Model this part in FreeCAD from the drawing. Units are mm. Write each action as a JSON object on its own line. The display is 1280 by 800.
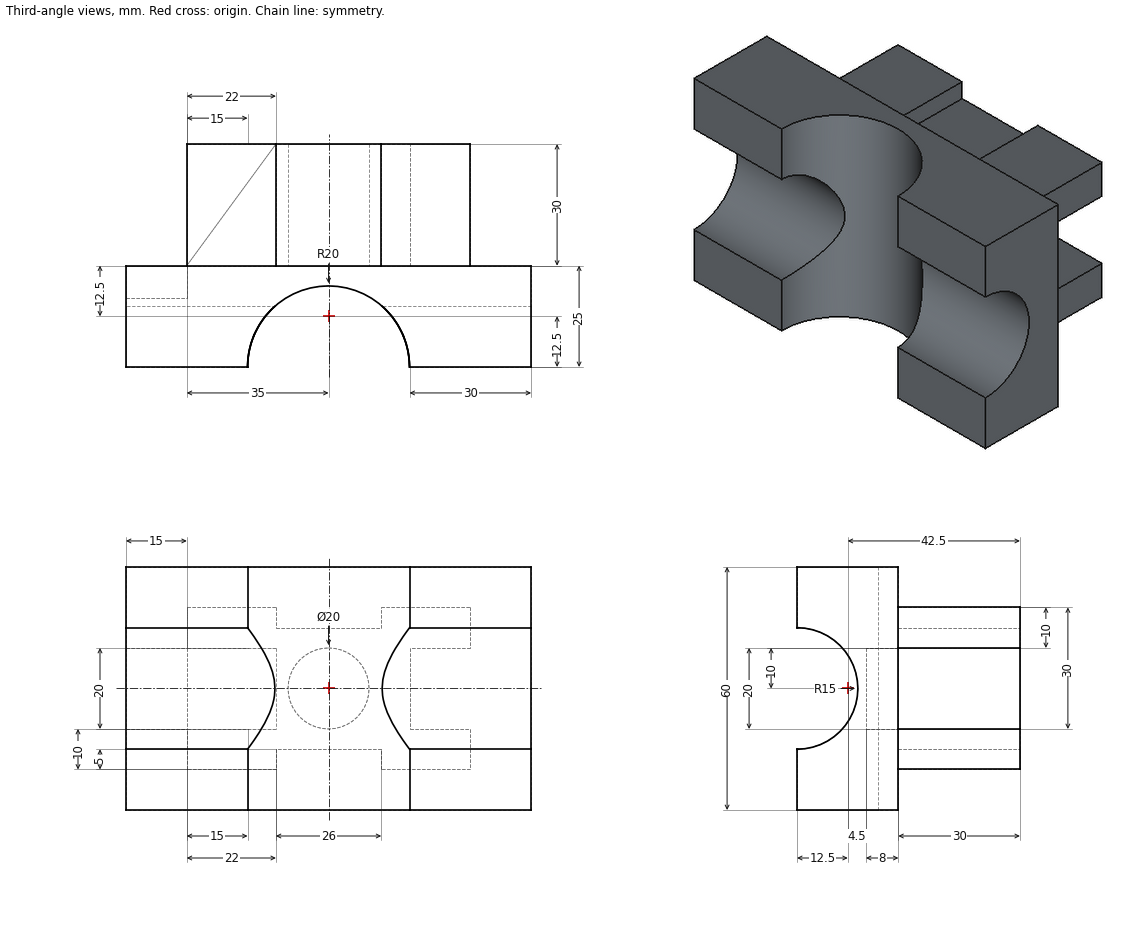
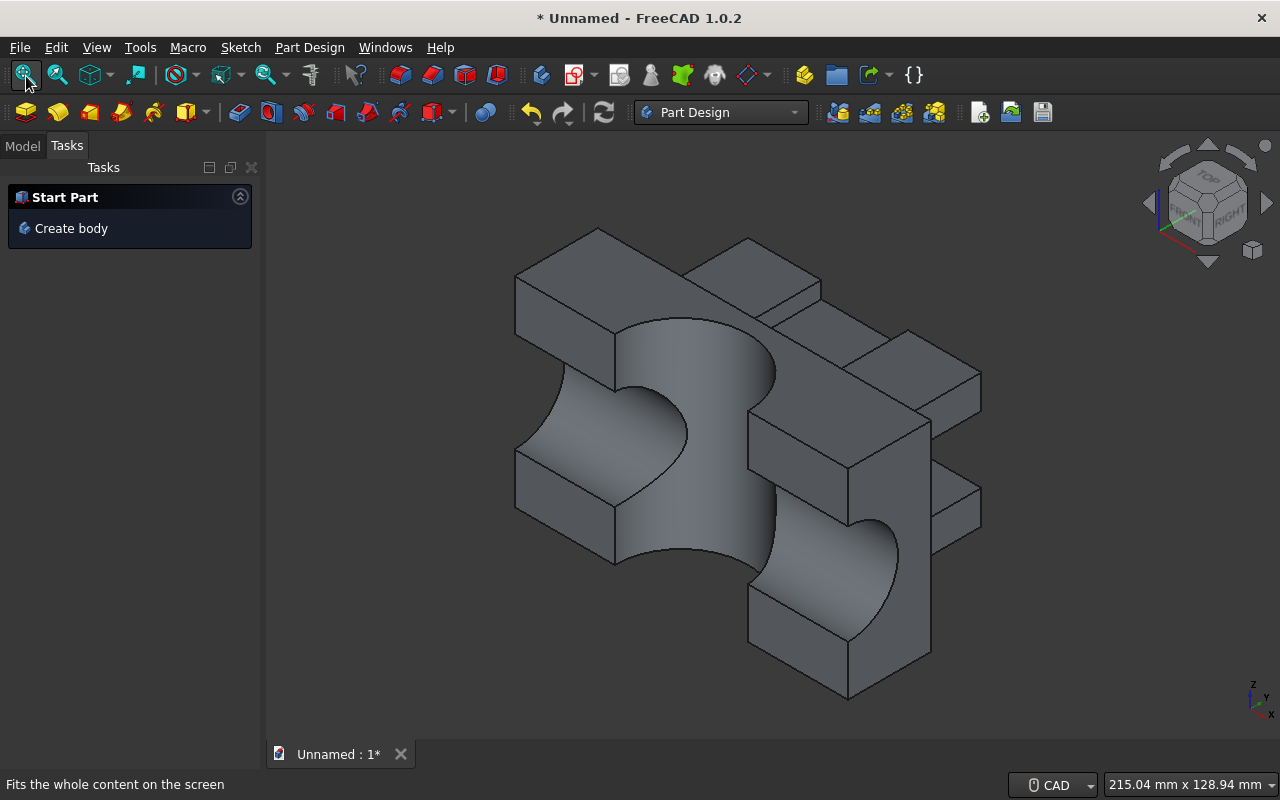
{"action": "left_click", "coordinate": [735, 287]}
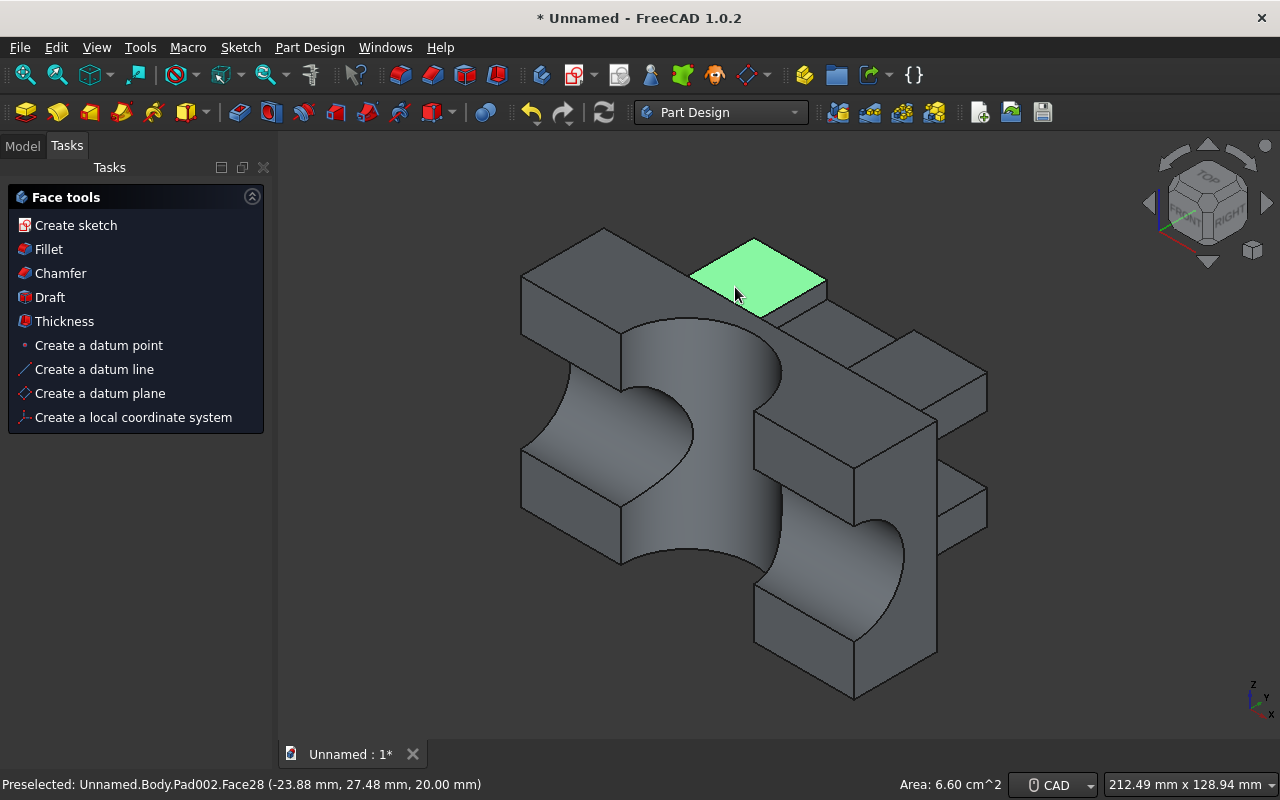
{"action": "left_click", "coordinate": [574, 76]}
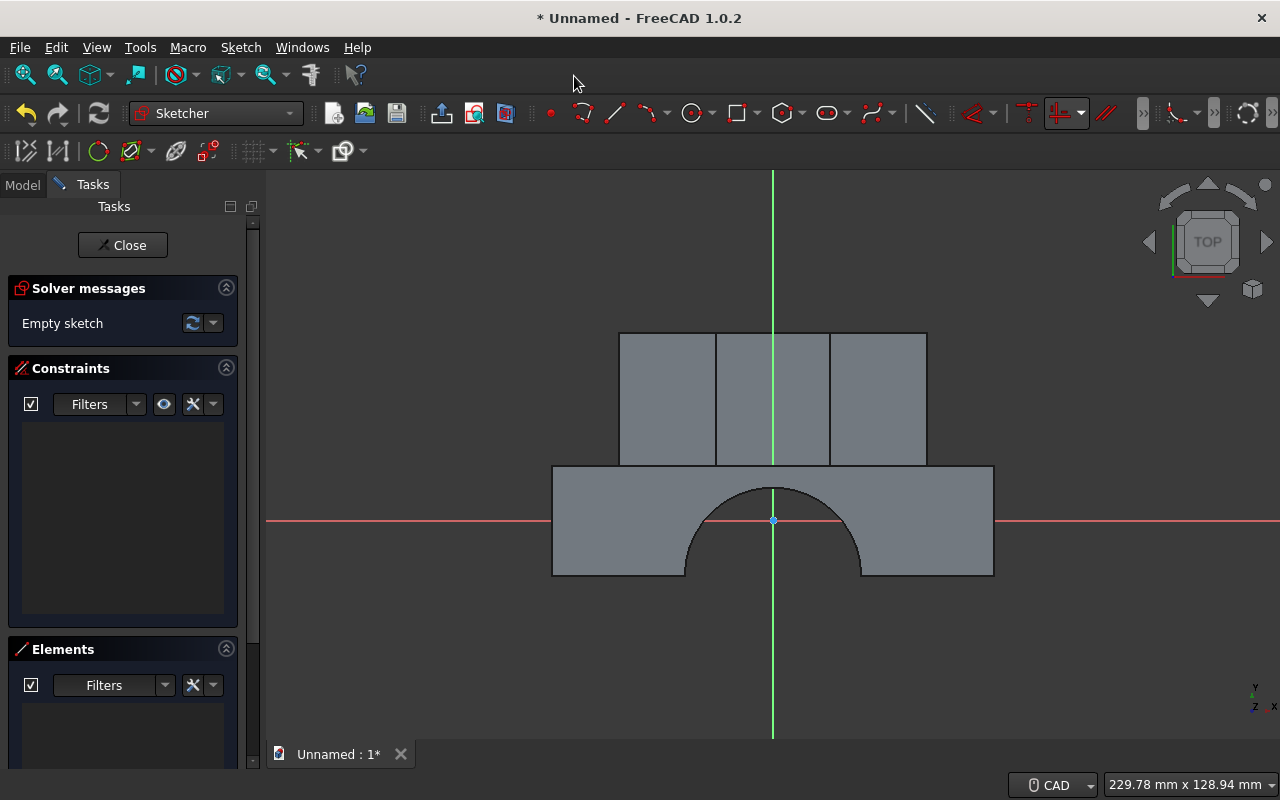
{"action": "key", "text": "q s"}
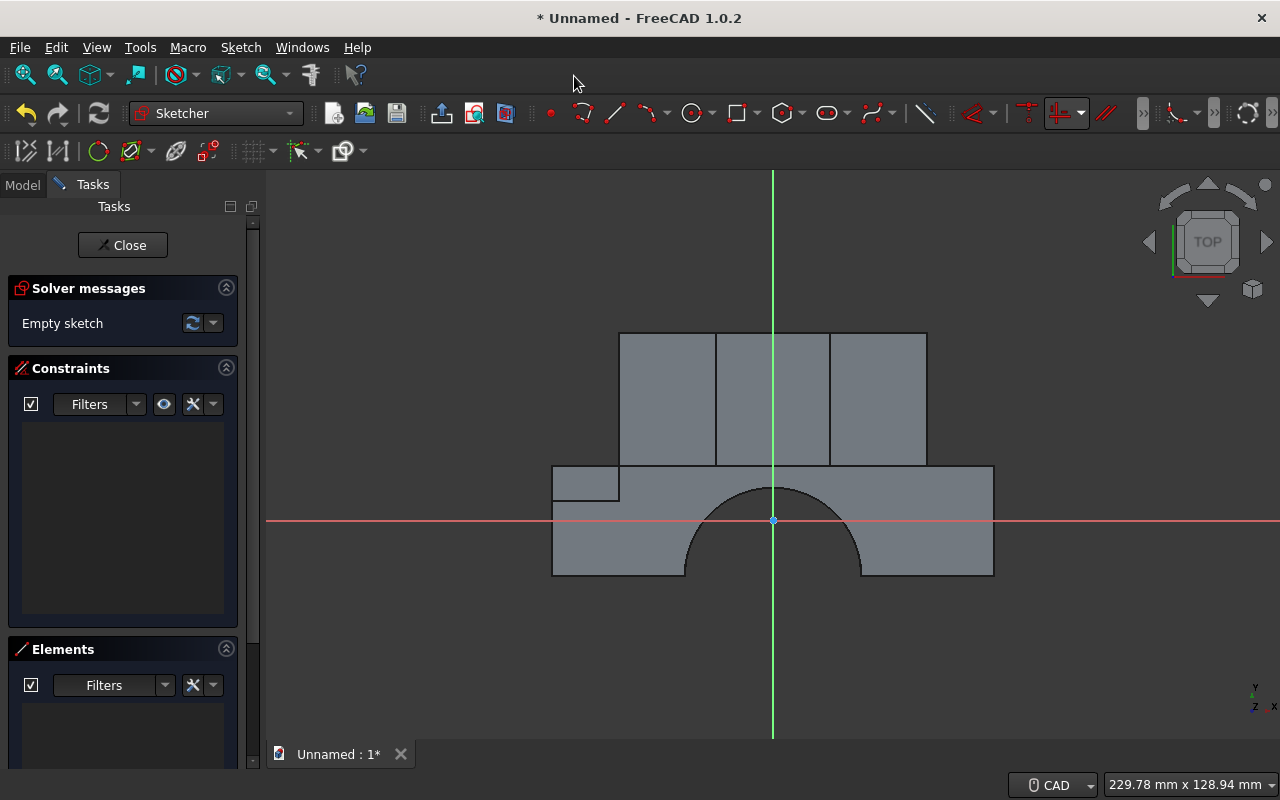
{"action": "scroll", "coordinate": [685, 393], "scroll_direction": "up", "scroll_amount": 3}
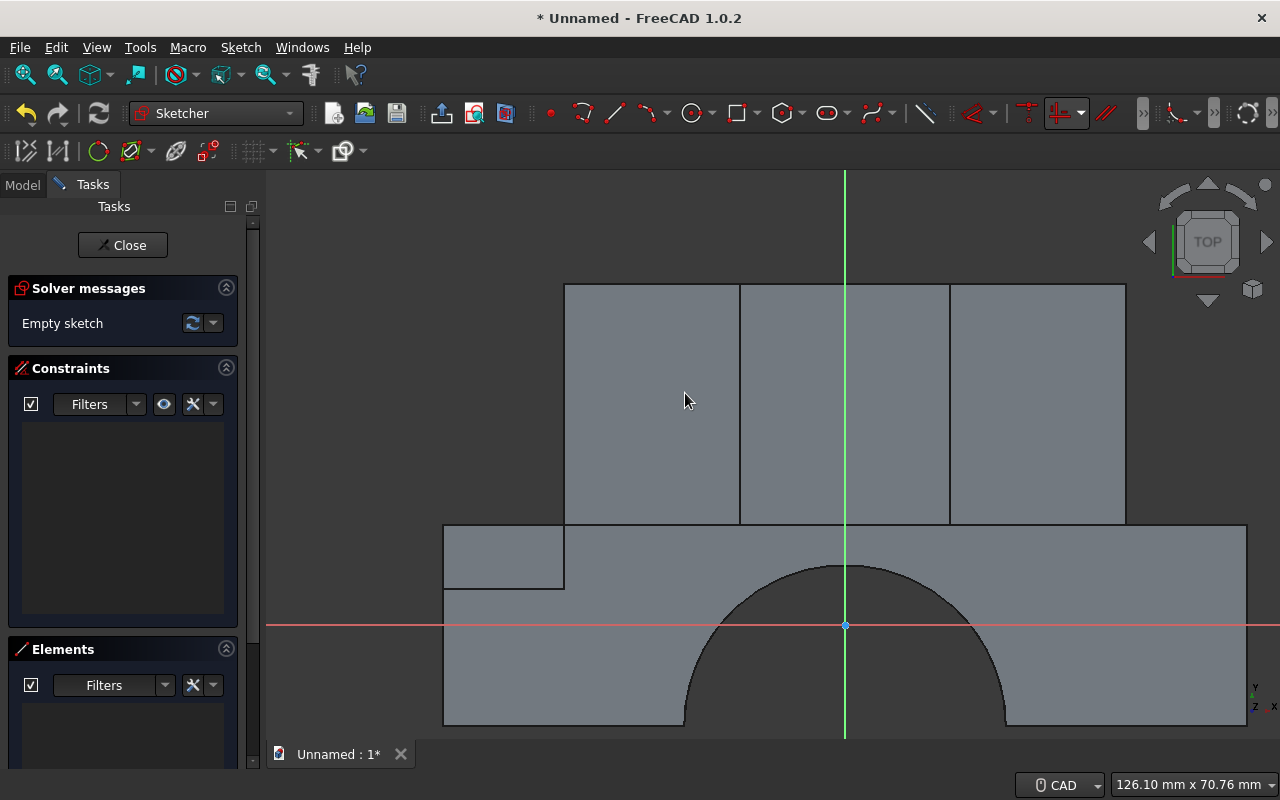
{"action": "left_click", "coordinate": [584, 114]}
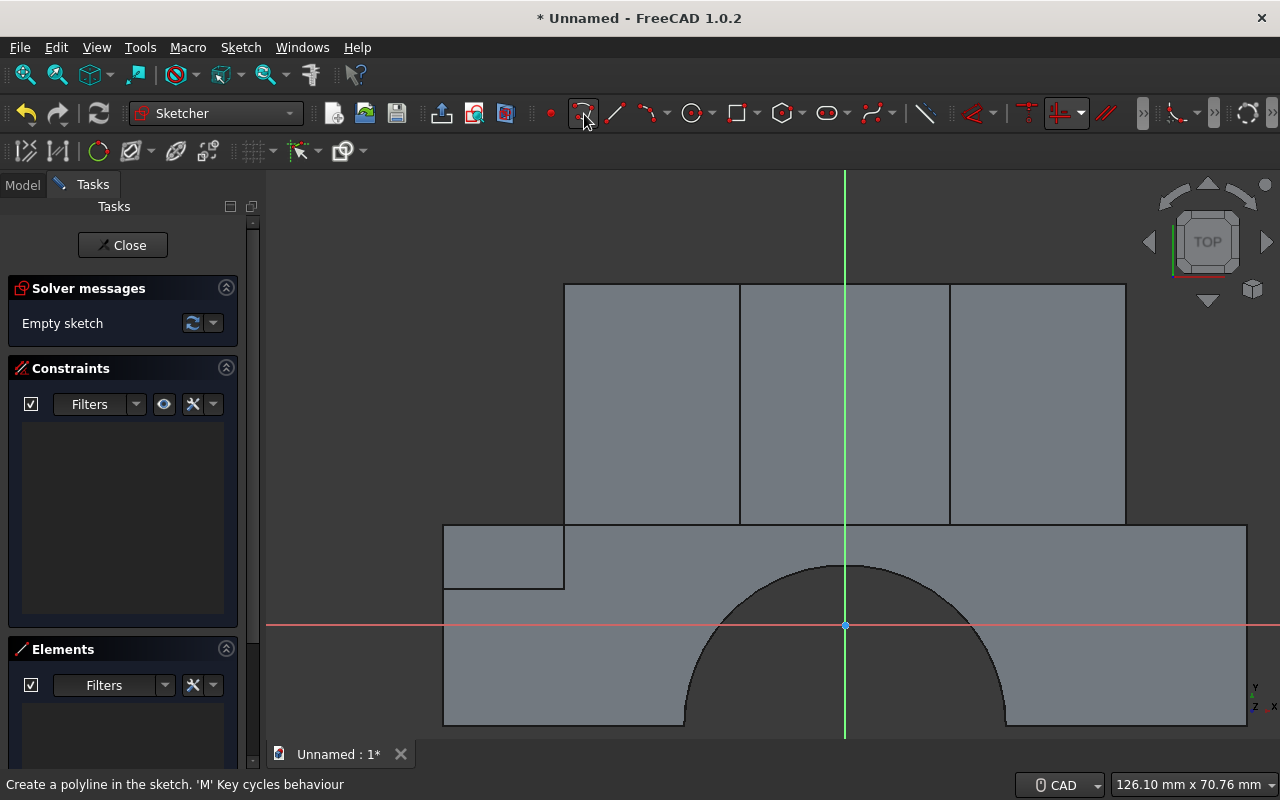
{"action": "left_click", "coordinate": [564, 525]}
{"action": "left_click", "coordinate": [740, 284]}
{"action": "left_click", "coordinate": [564, 284]}
{"action": "left_click", "coordinate": [564, 526]}
{"action": "key", "text": "Escape"}
{"action": "key", "text": "Escape"}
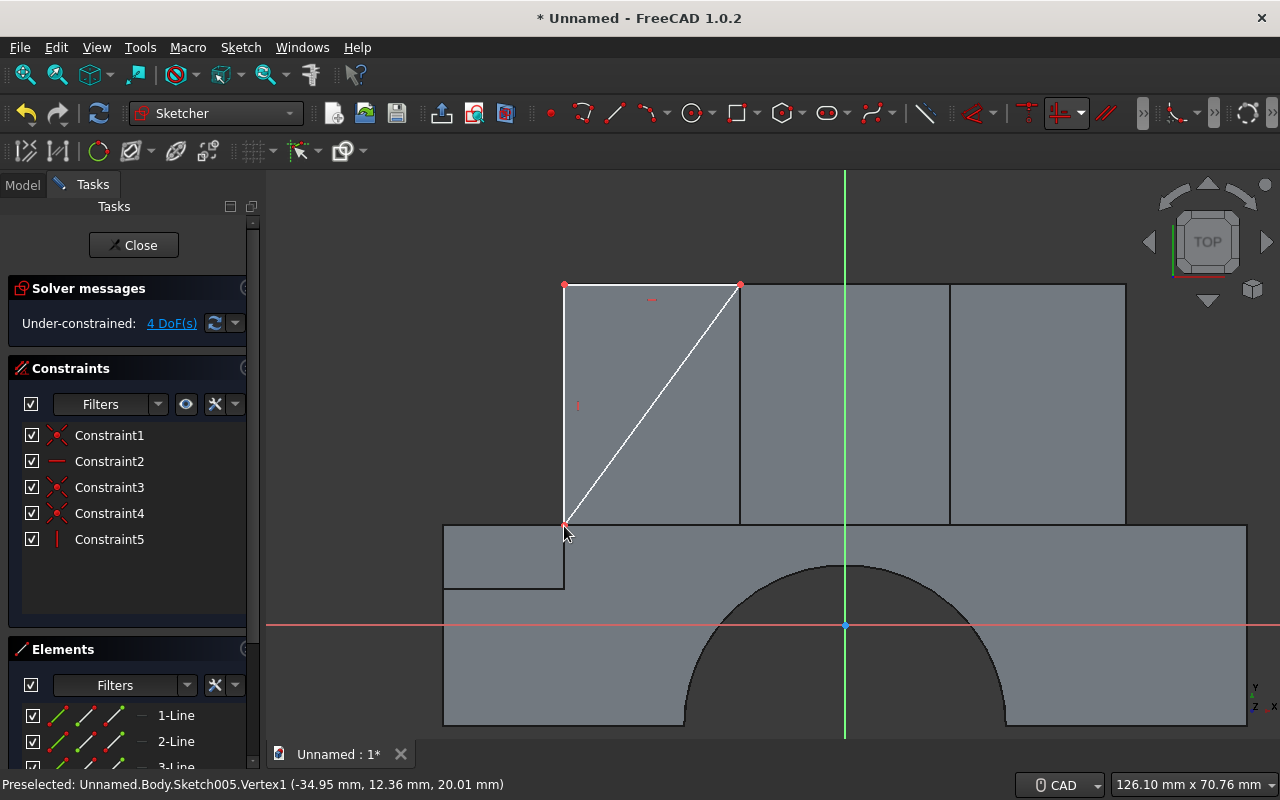
{"action": "left_click", "coordinate": [972, 114]}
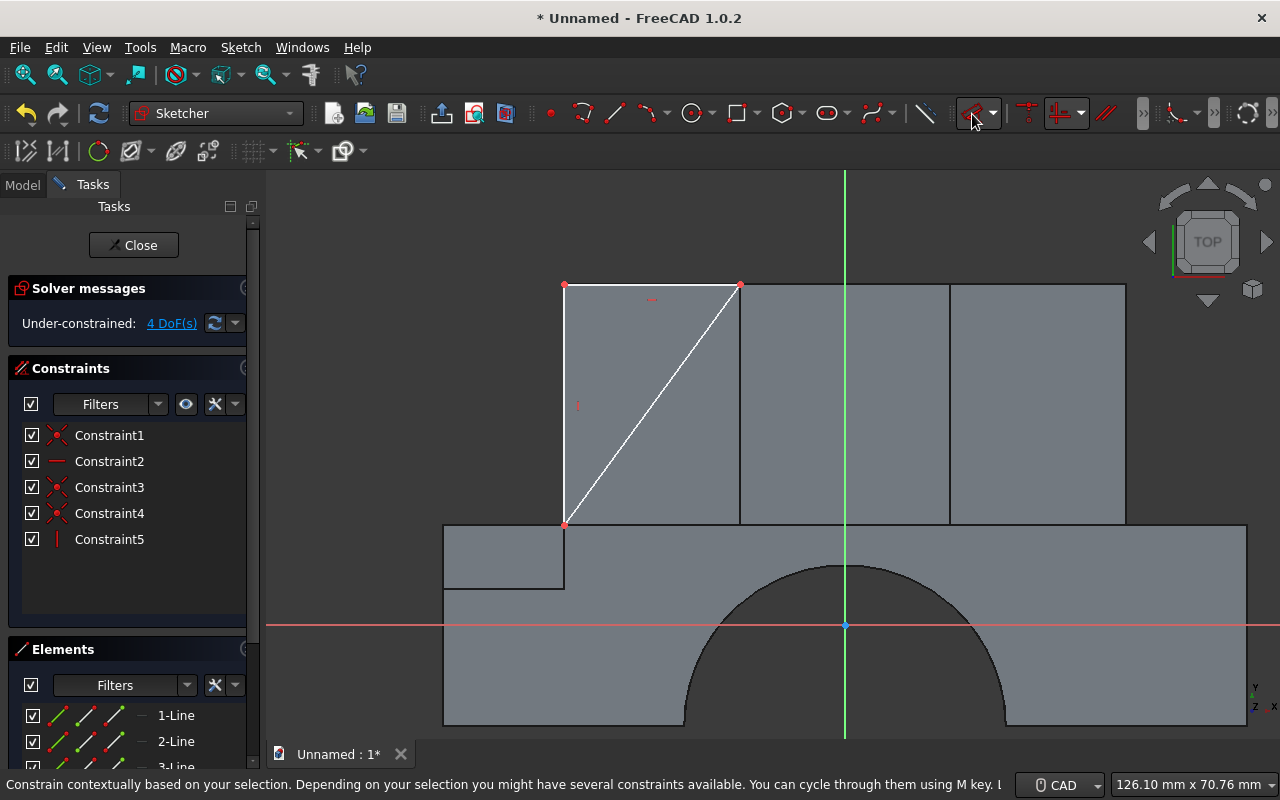
{"action": "left_click", "coordinate": [687, 285]}
{"action": "left_click", "coordinate": [652, 251]}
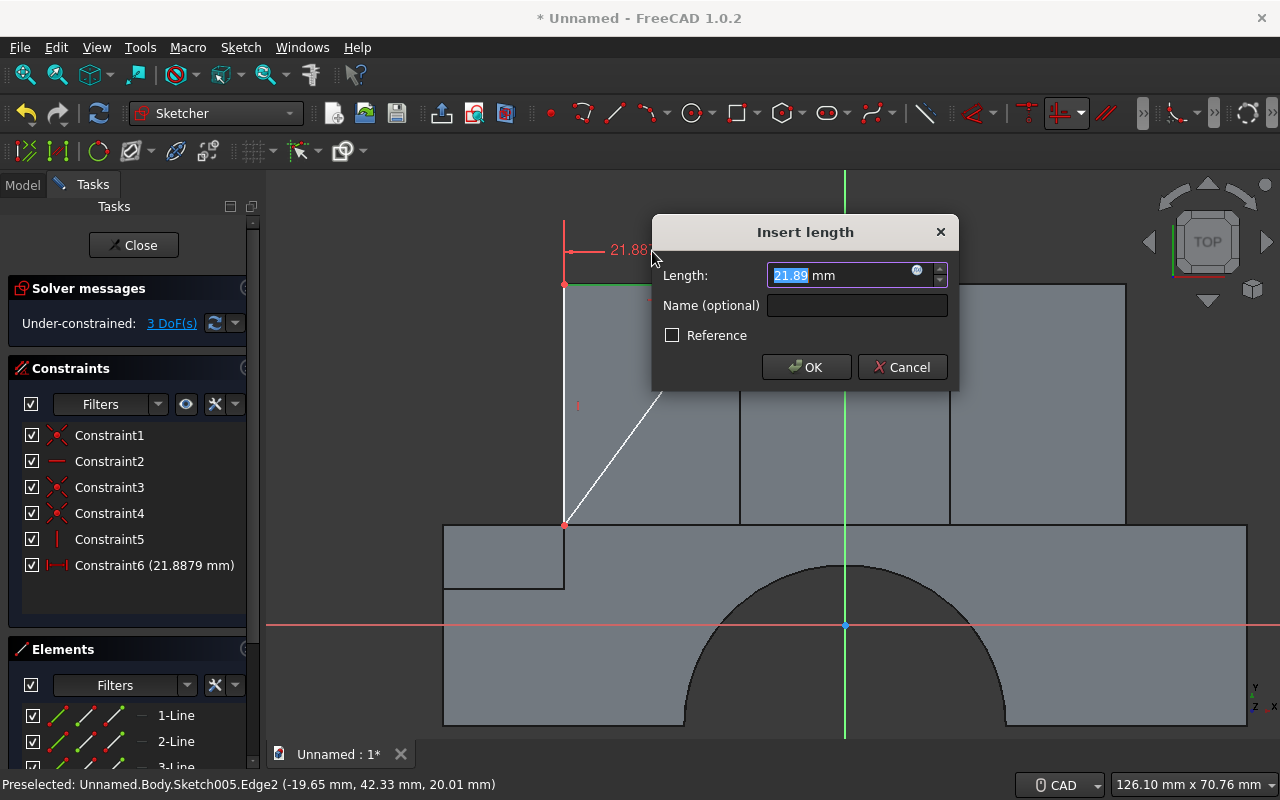
{"action": "type", "text": "22"}
{"action": "key", "text": "Return"}